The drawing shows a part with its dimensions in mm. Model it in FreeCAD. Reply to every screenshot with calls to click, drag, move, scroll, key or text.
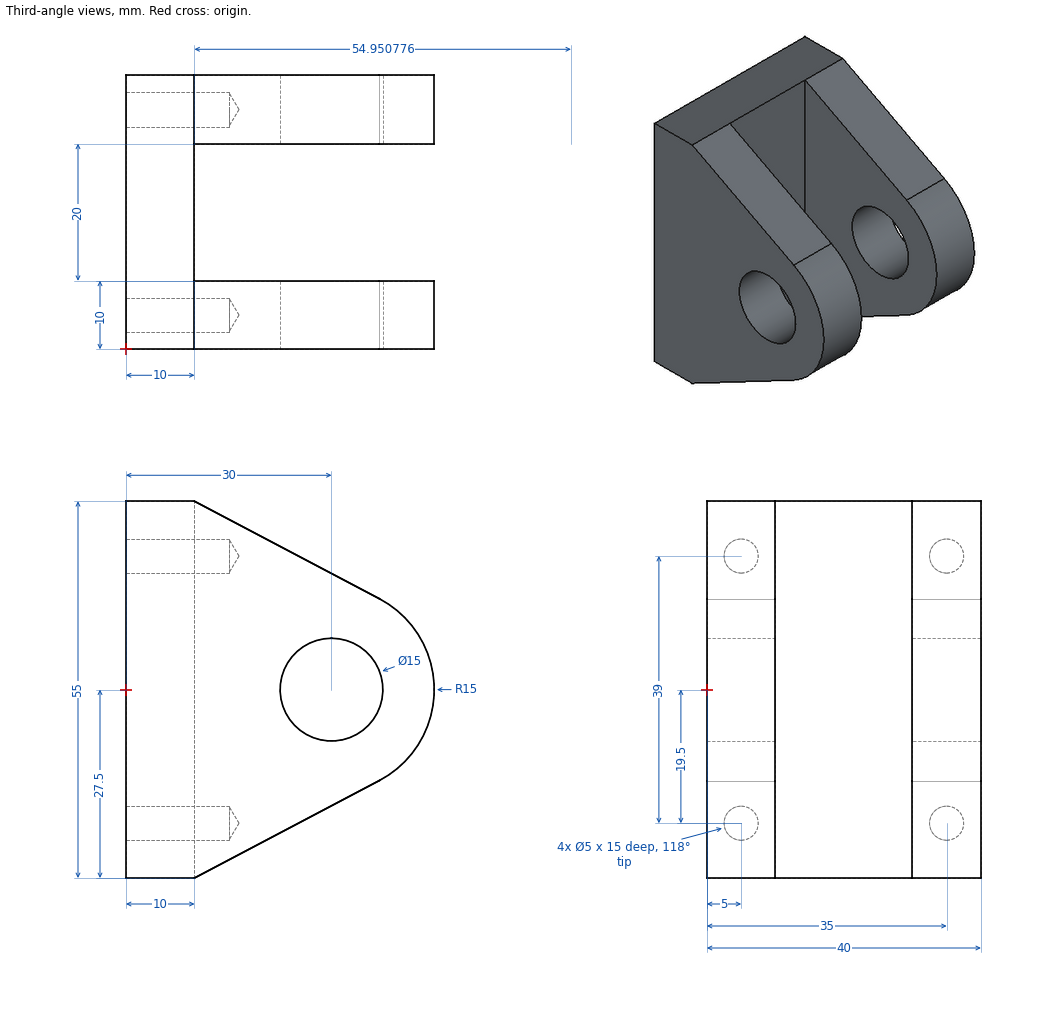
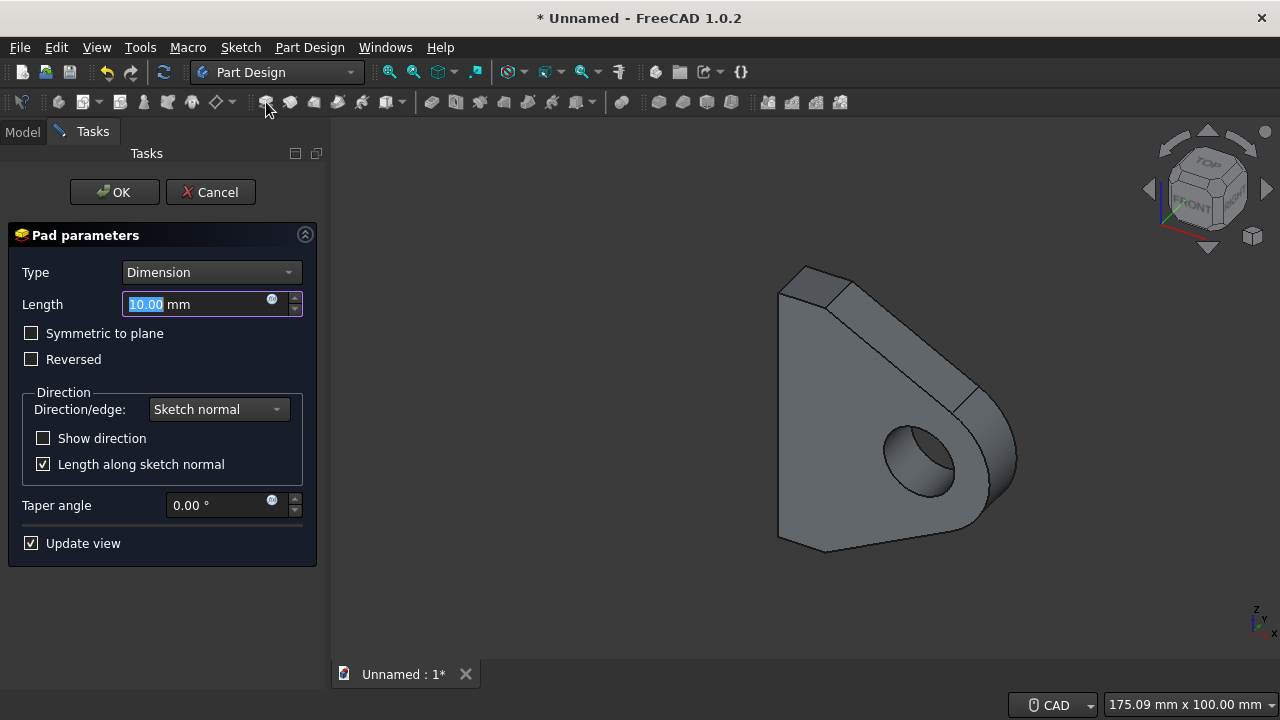
text(40)
key(Tab)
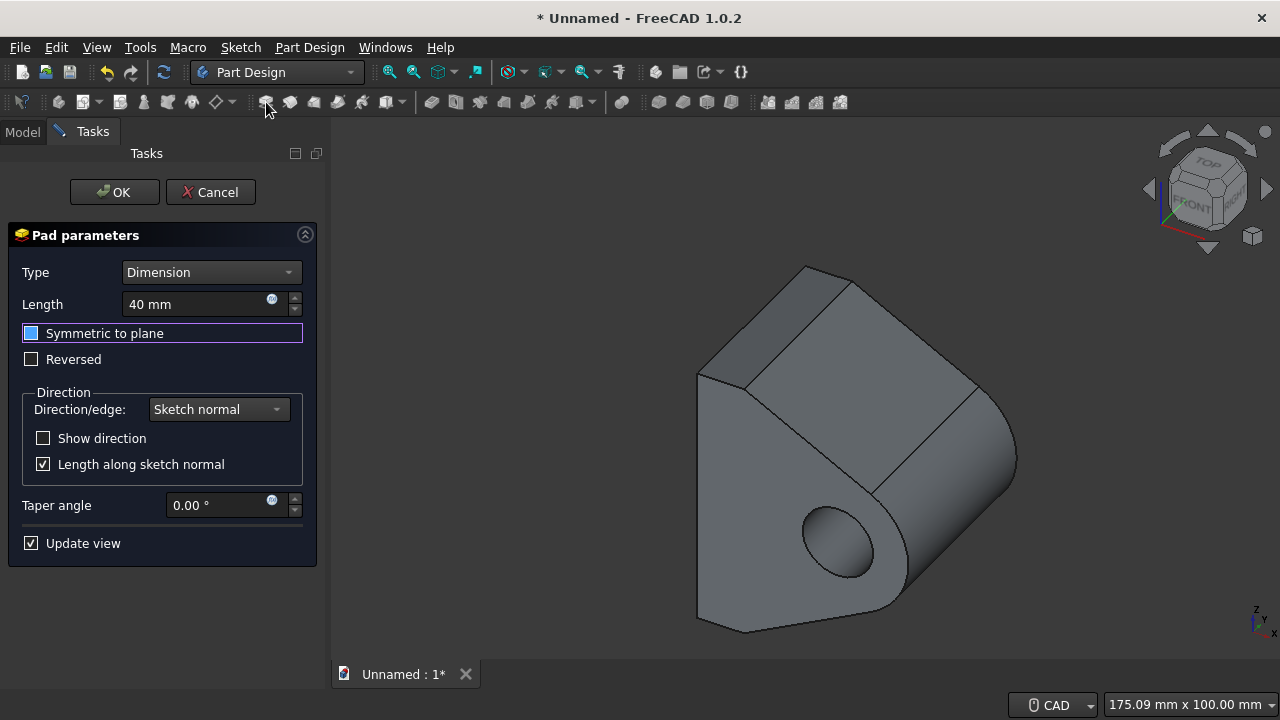
click(30, 359)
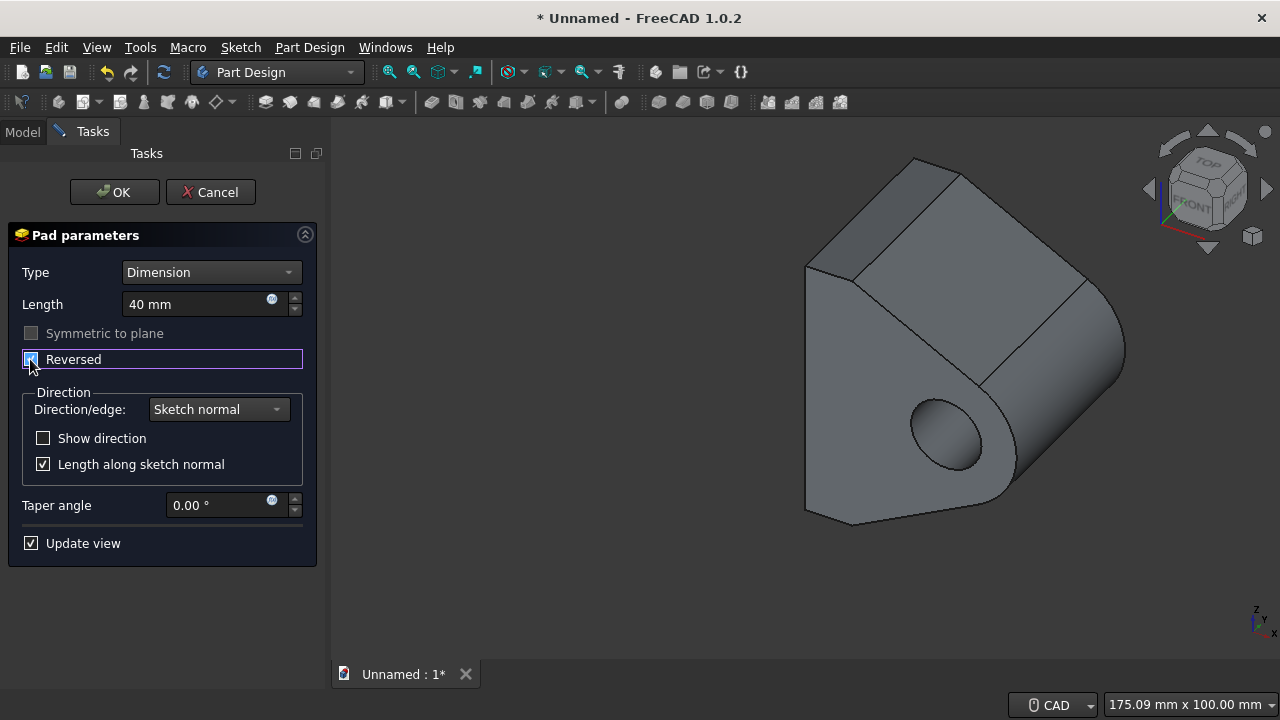
click(115, 192)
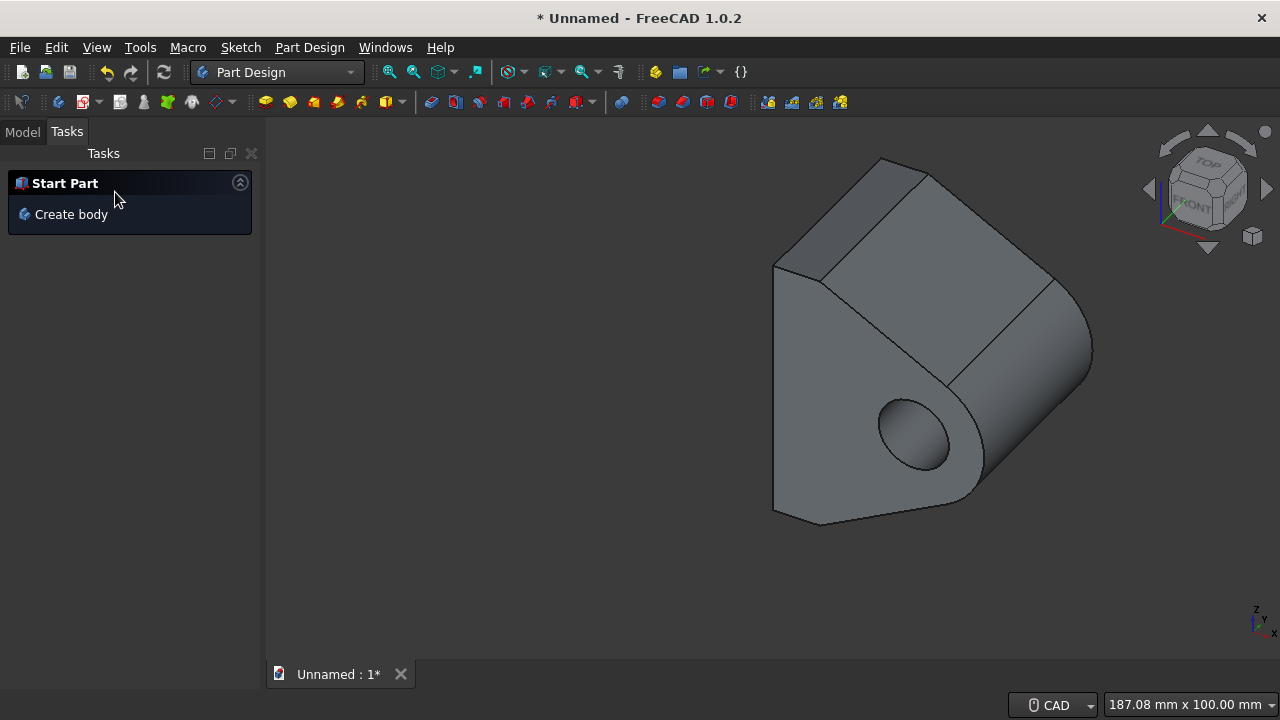
key(5)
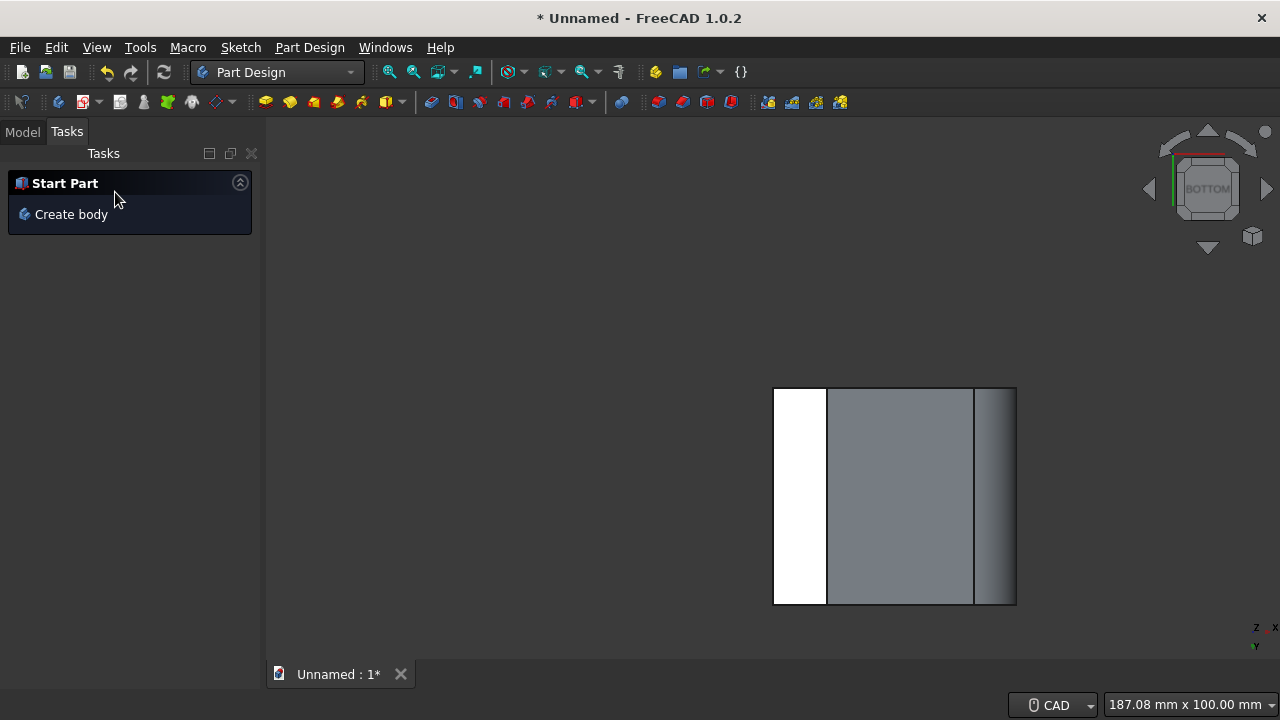
key(v)
key(f)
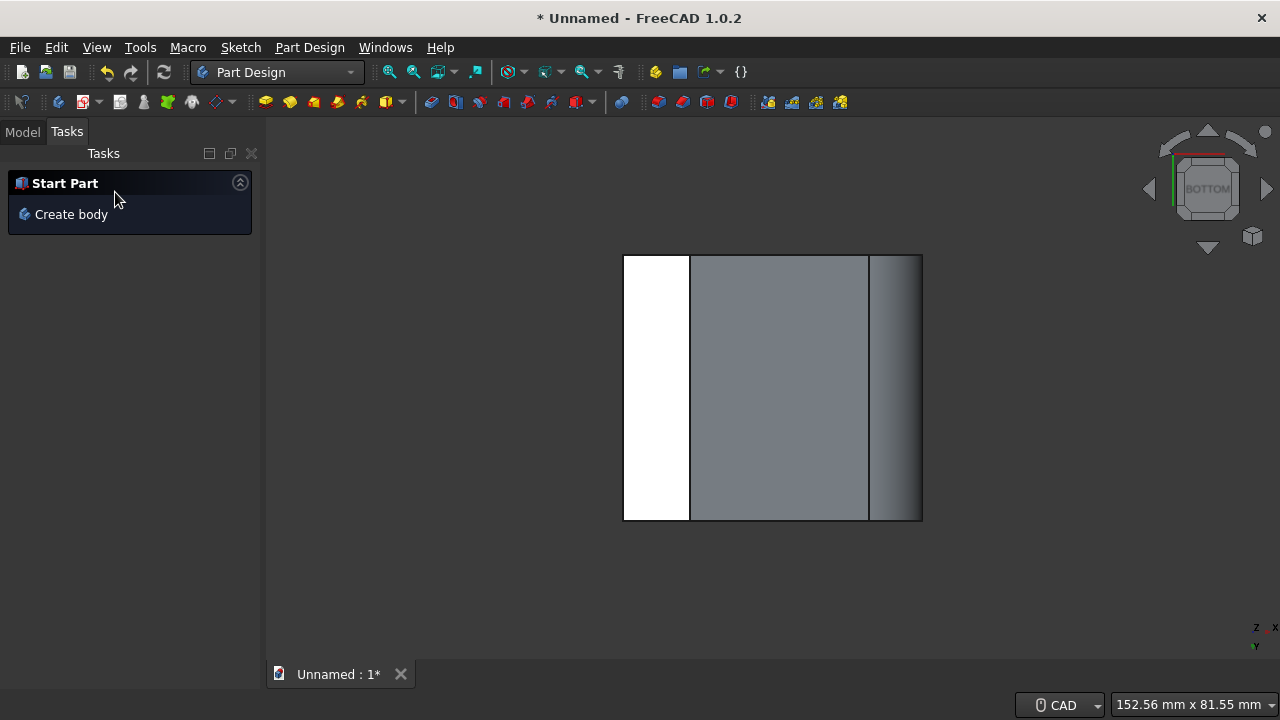
click(657, 463)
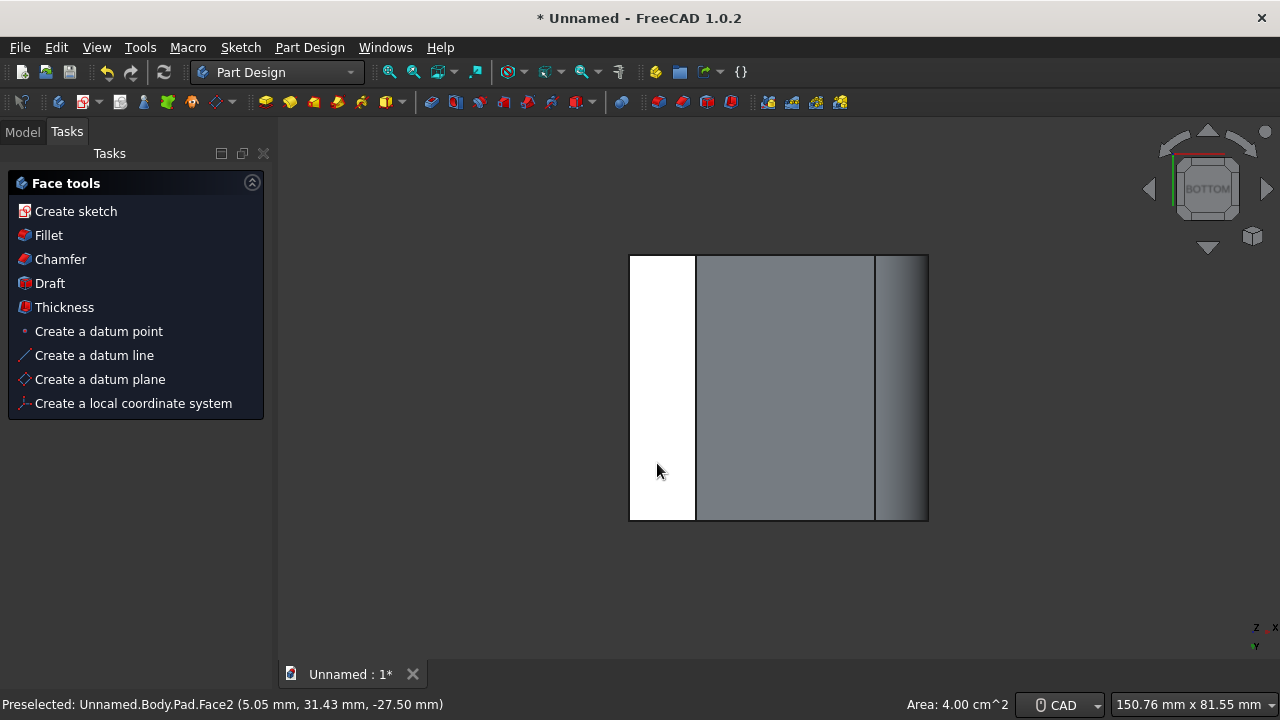
click(84, 102)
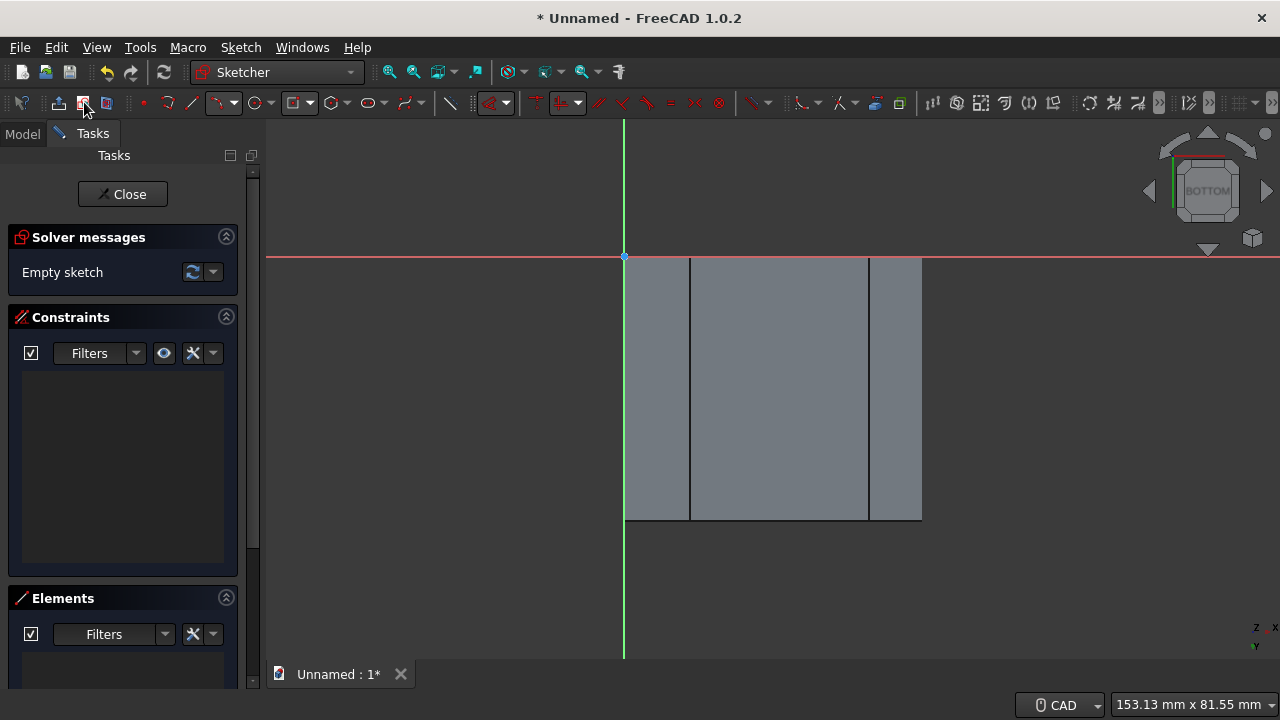
click(312, 104)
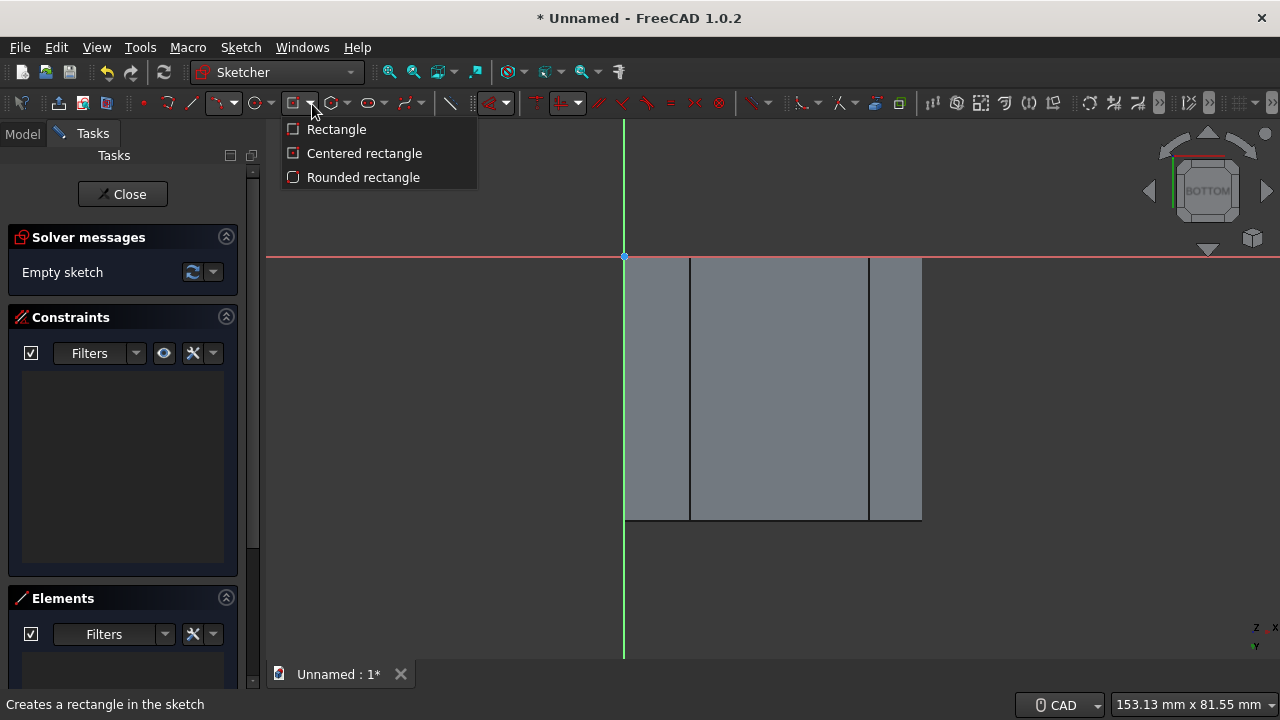
click(380, 129)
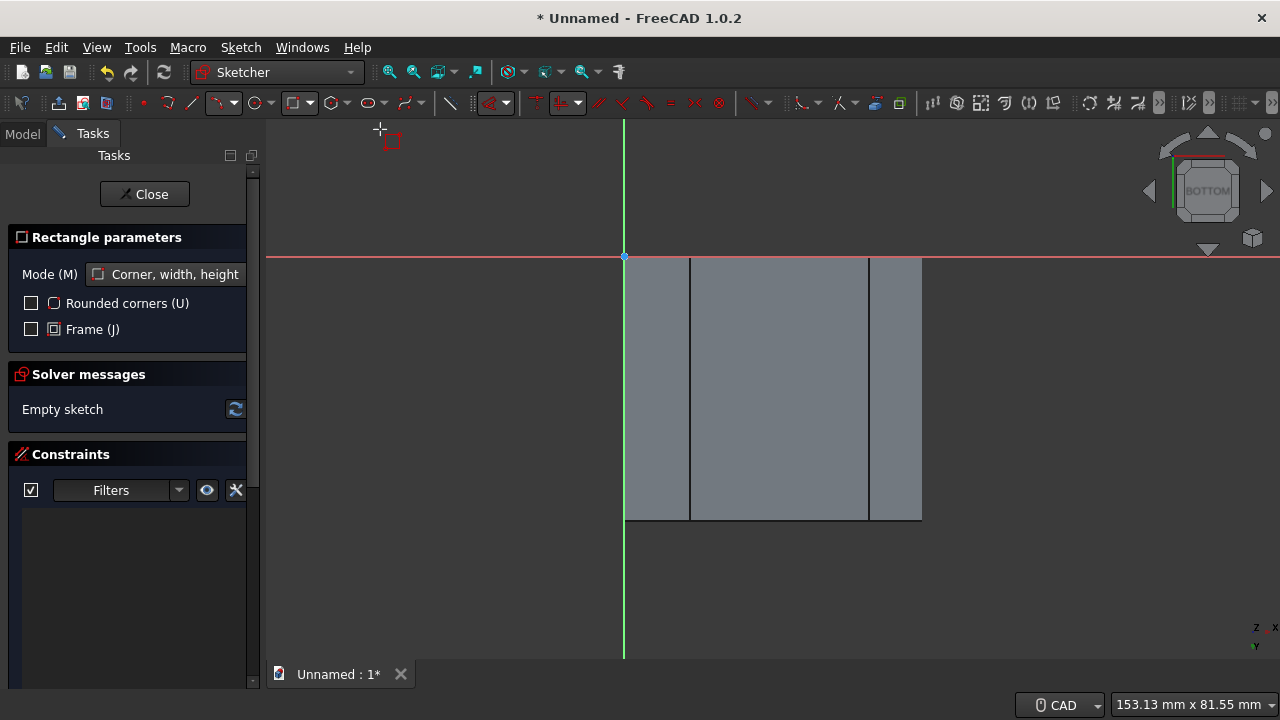
click(690, 323)
click(1054, 455)
key(Escape)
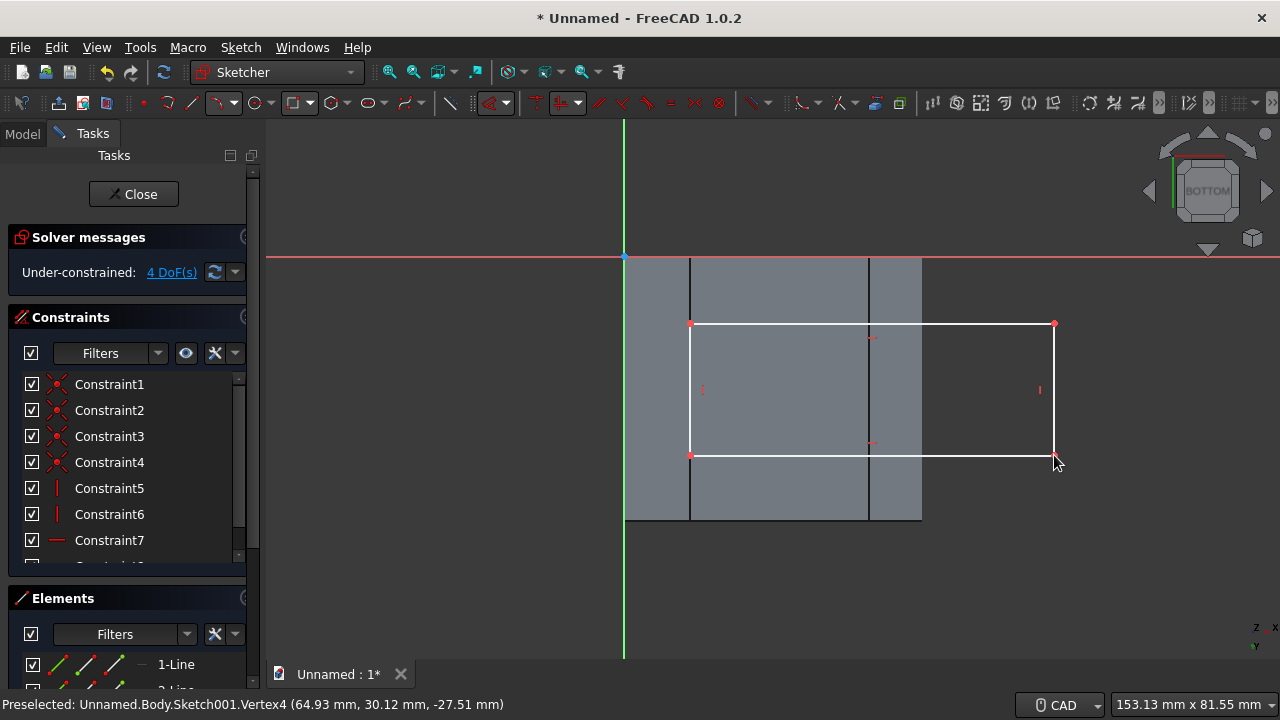
click(690, 364)